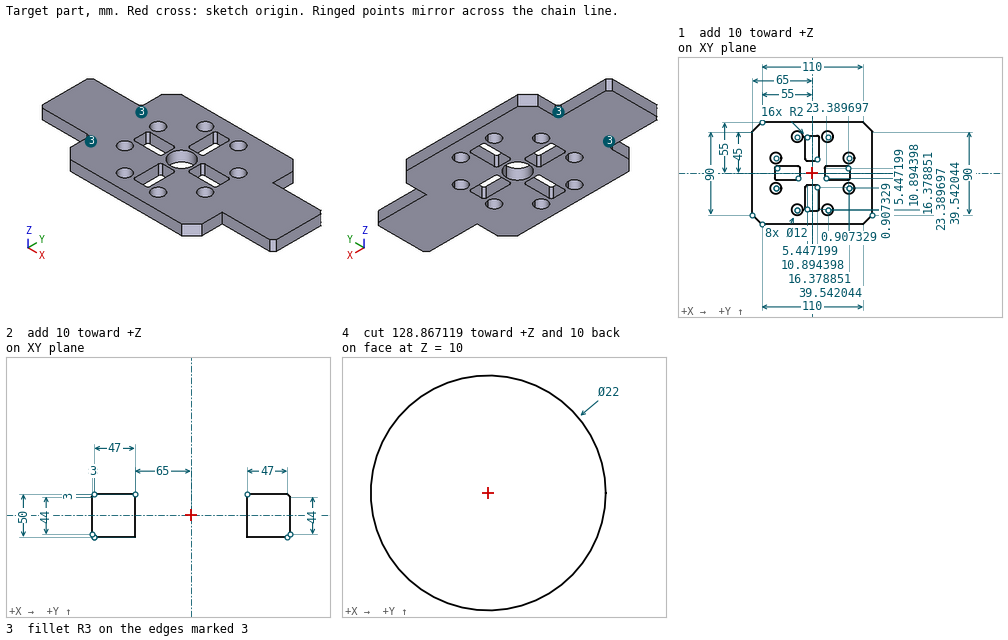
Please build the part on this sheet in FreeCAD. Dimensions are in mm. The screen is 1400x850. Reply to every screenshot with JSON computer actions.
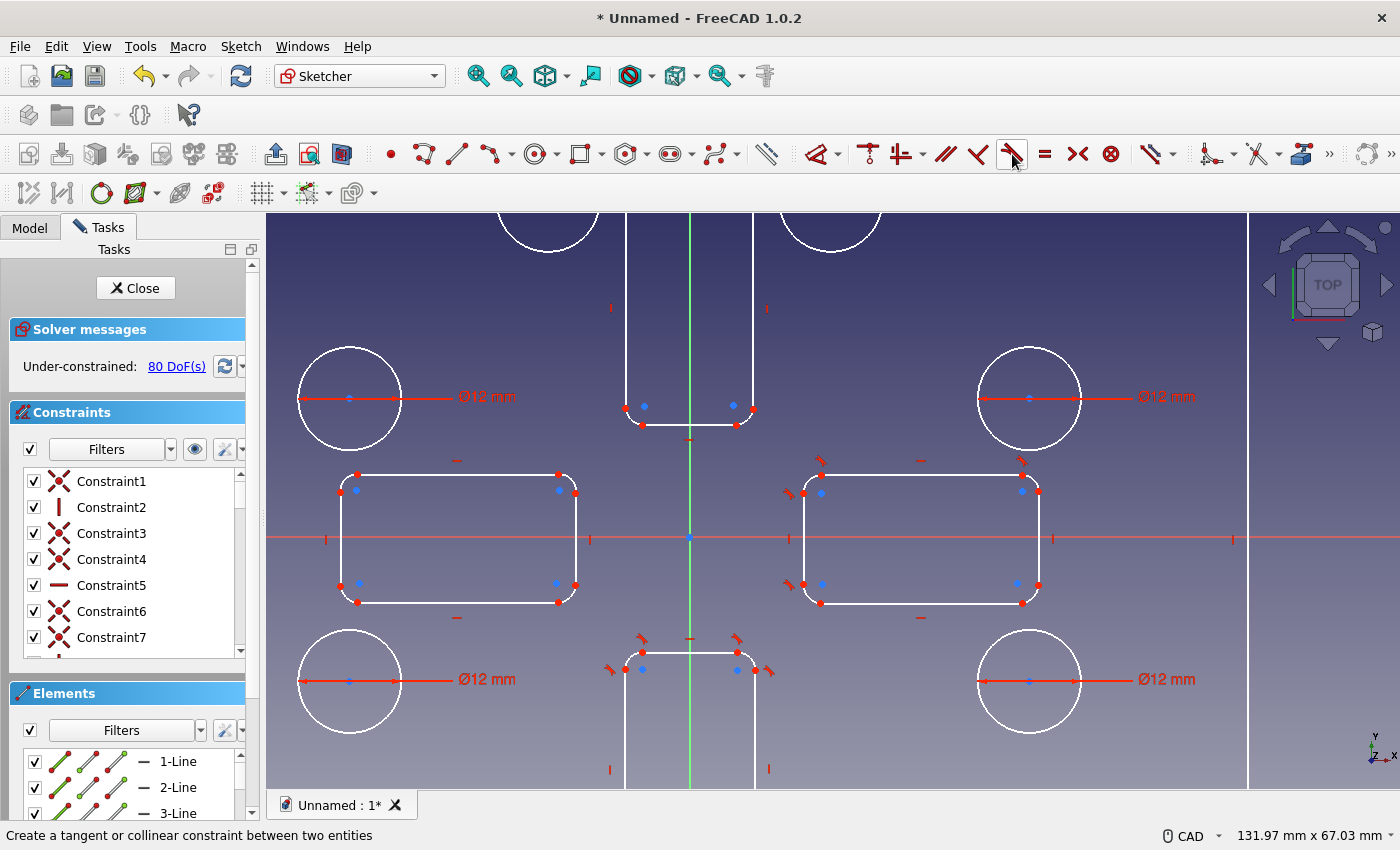
{"action": "left_click", "coordinate": [1039, 520]}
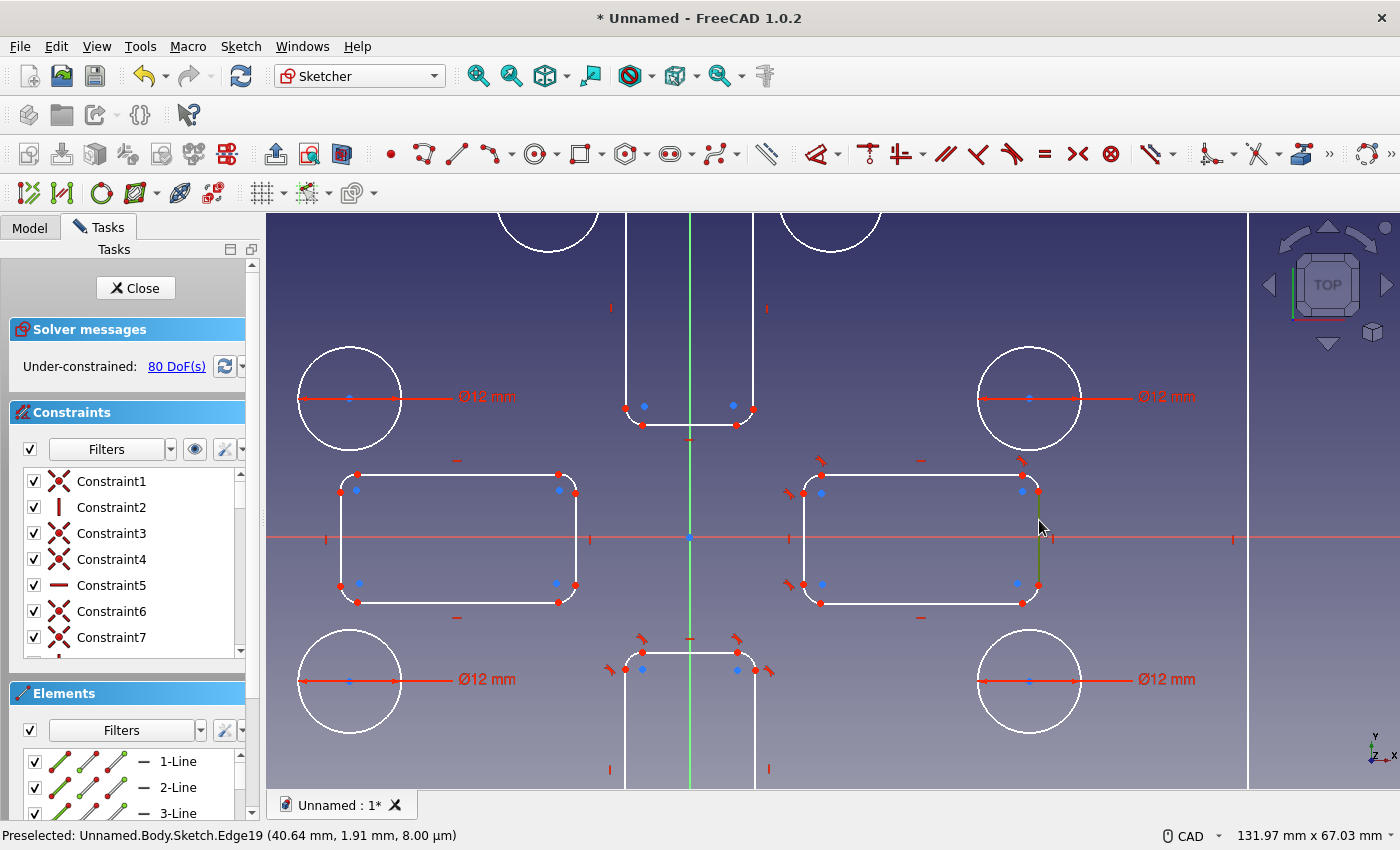
{"action": "left_click", "coordinate": [1034, 480]}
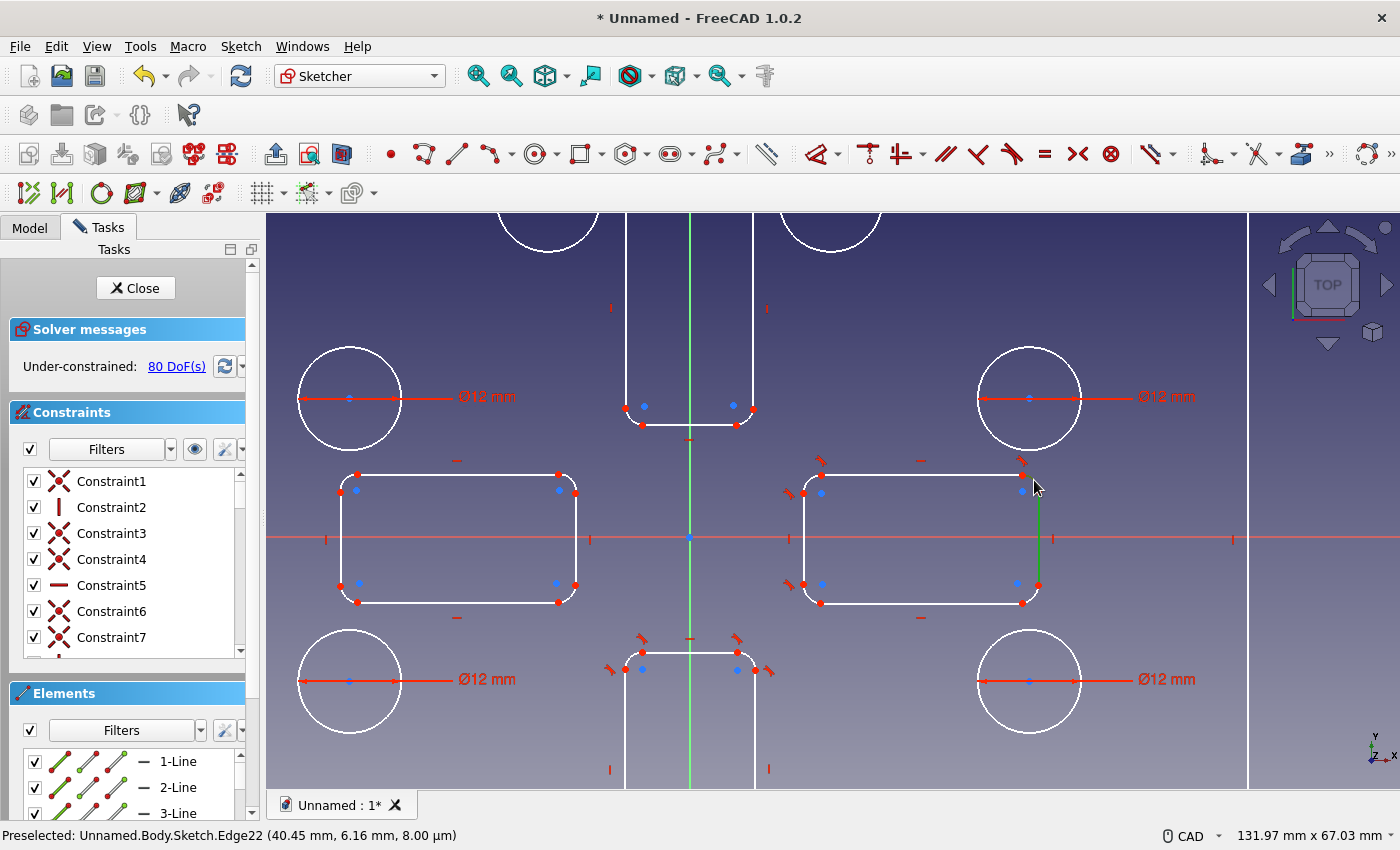
{"action": "left_click", "coordinate": [1012, 154]}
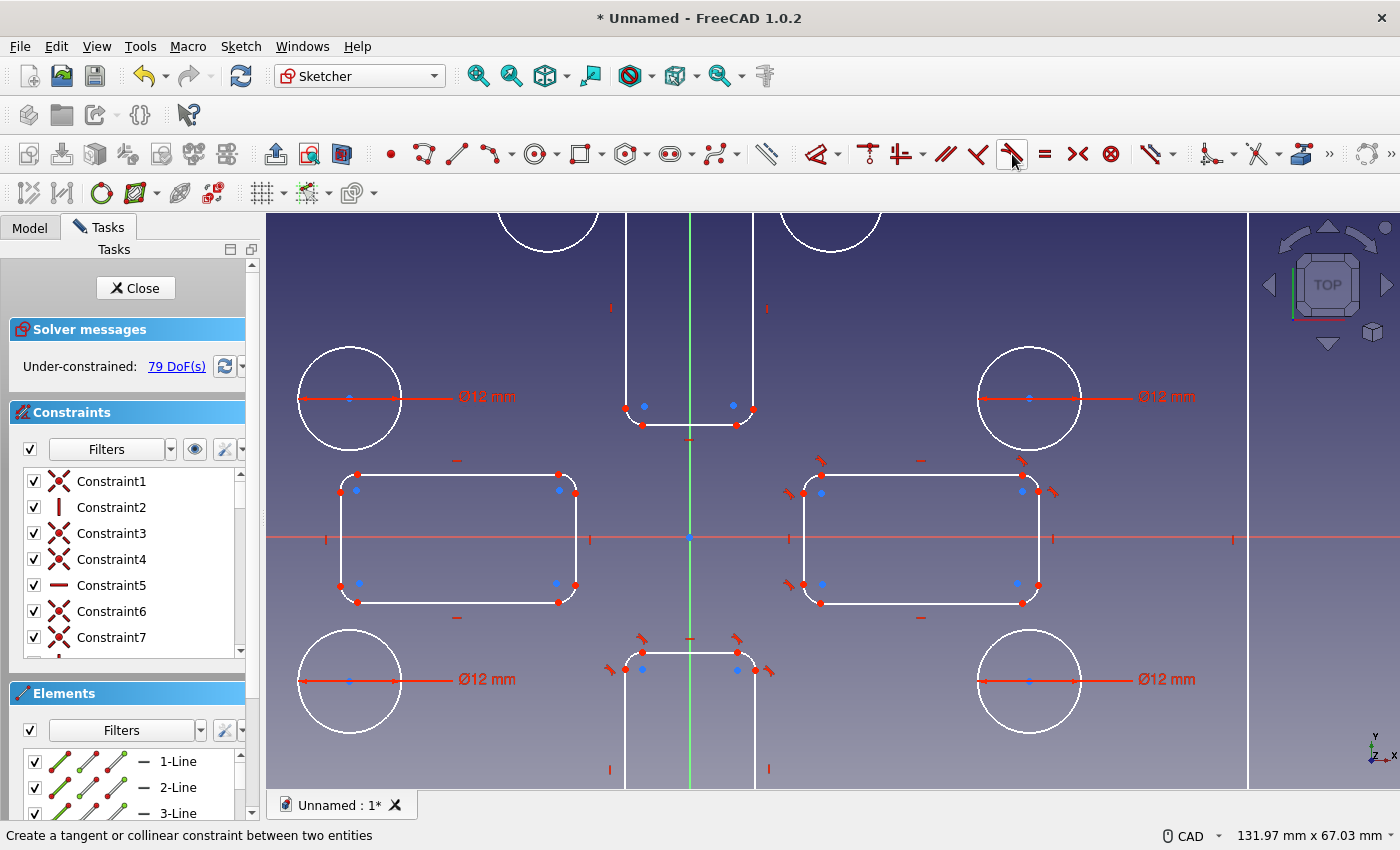
{"action": "left_click", "coordinate": [1039, 520]}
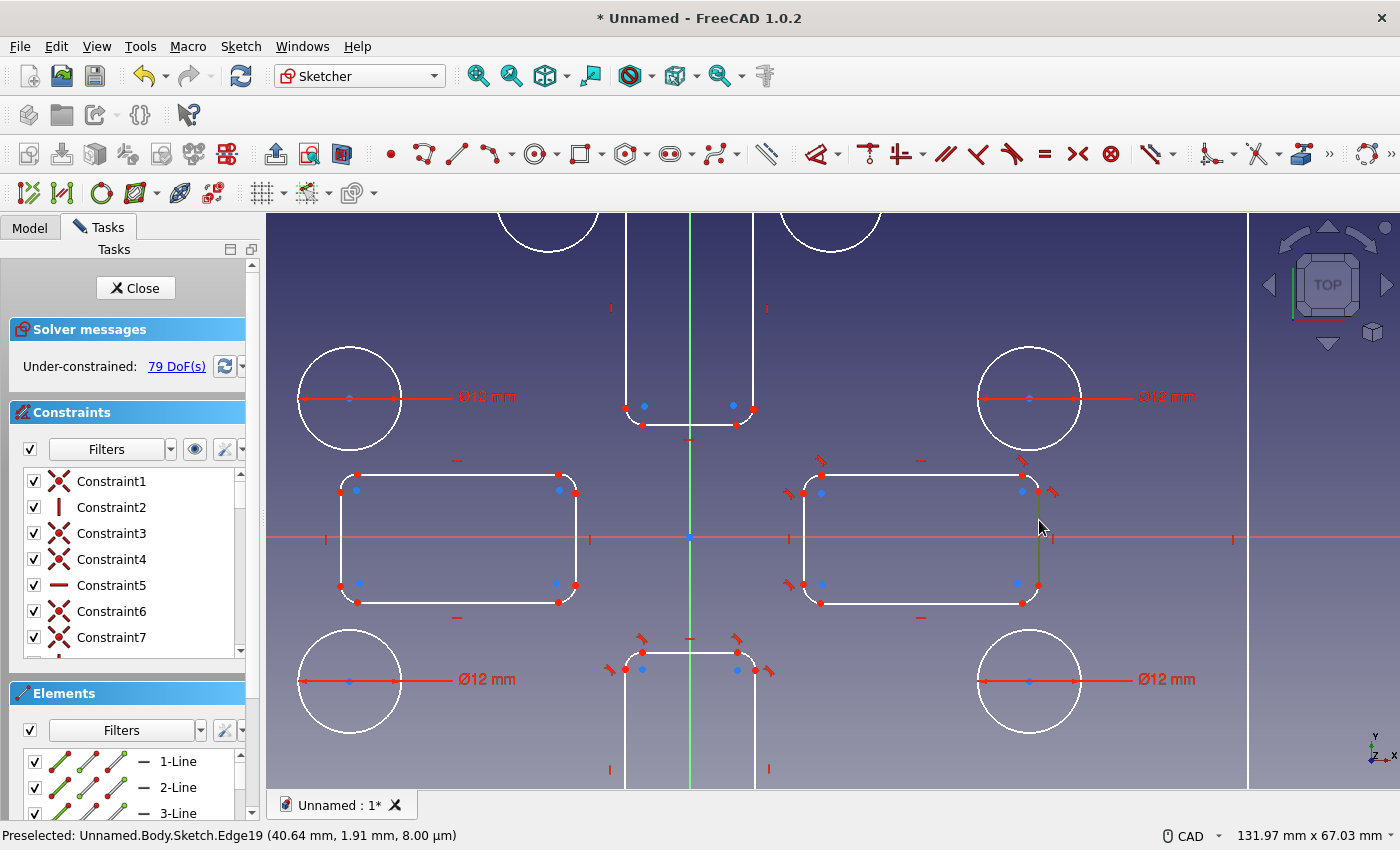
{"action": "left_click", "coordinate": [1033, 597]}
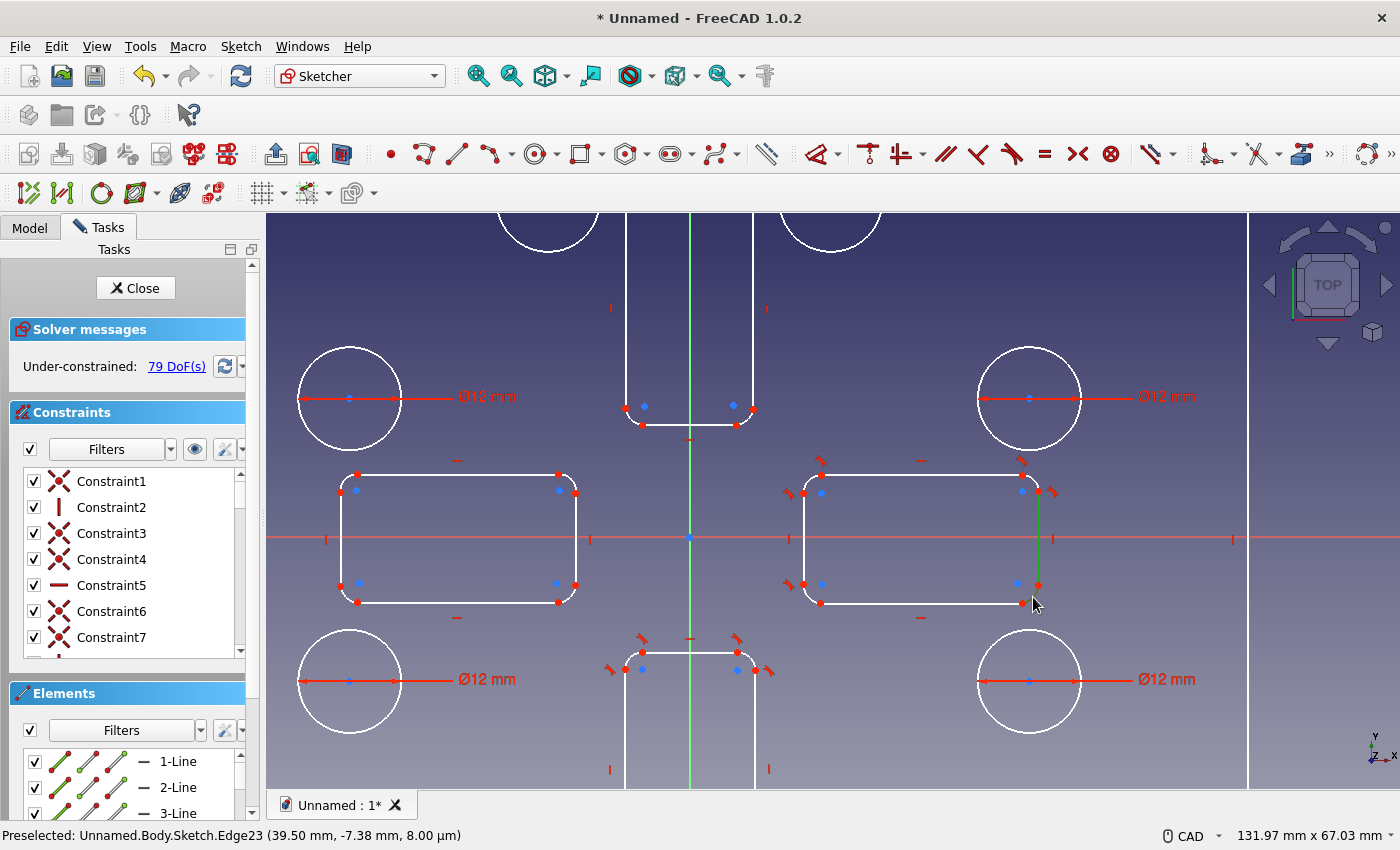
{"action": "left_click", "coordinate": [1012, 154]}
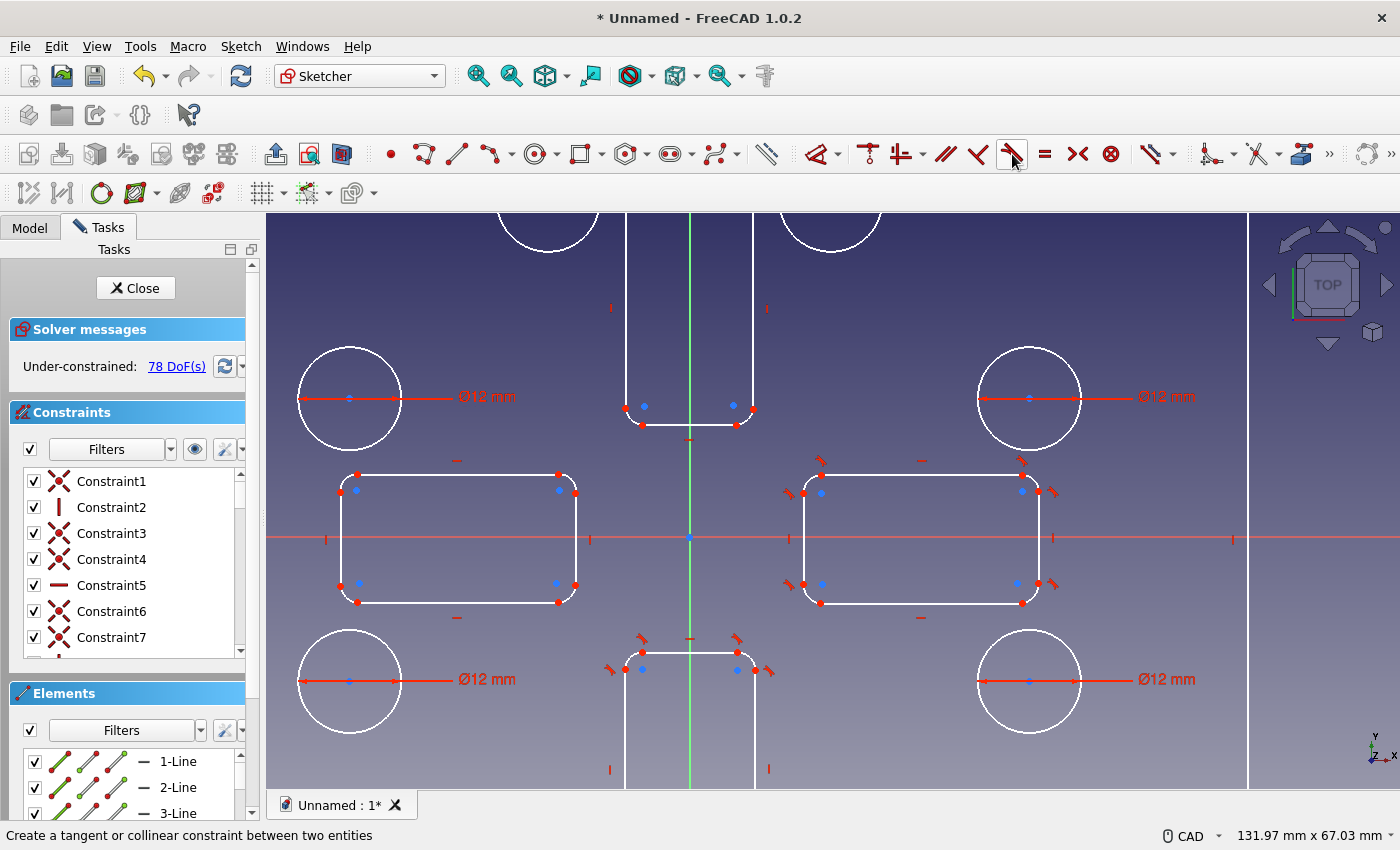
{"action": "left_click", "coordinate": [962, 604]}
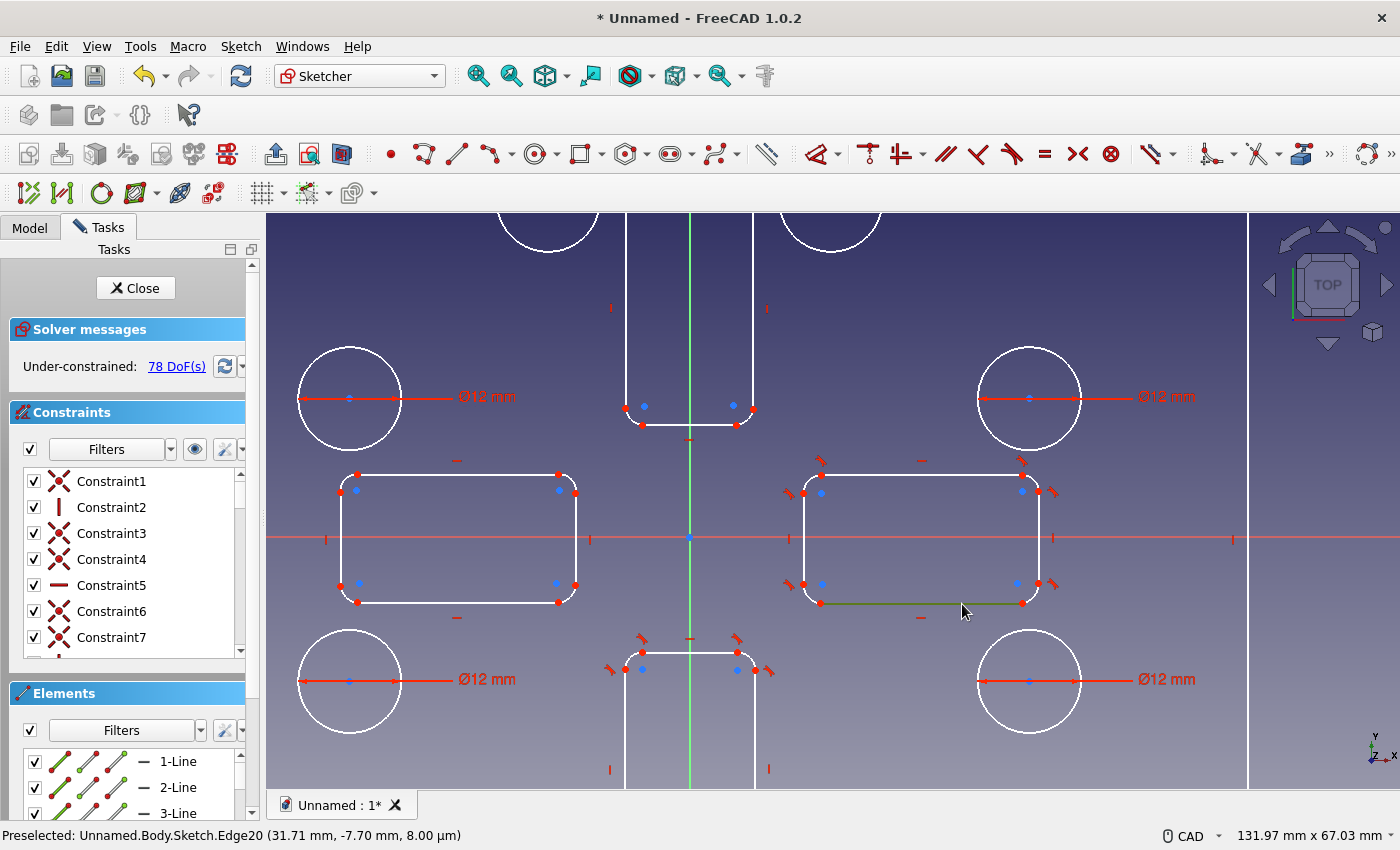
{"action": "left_click", "coordinate": [1034, 596]}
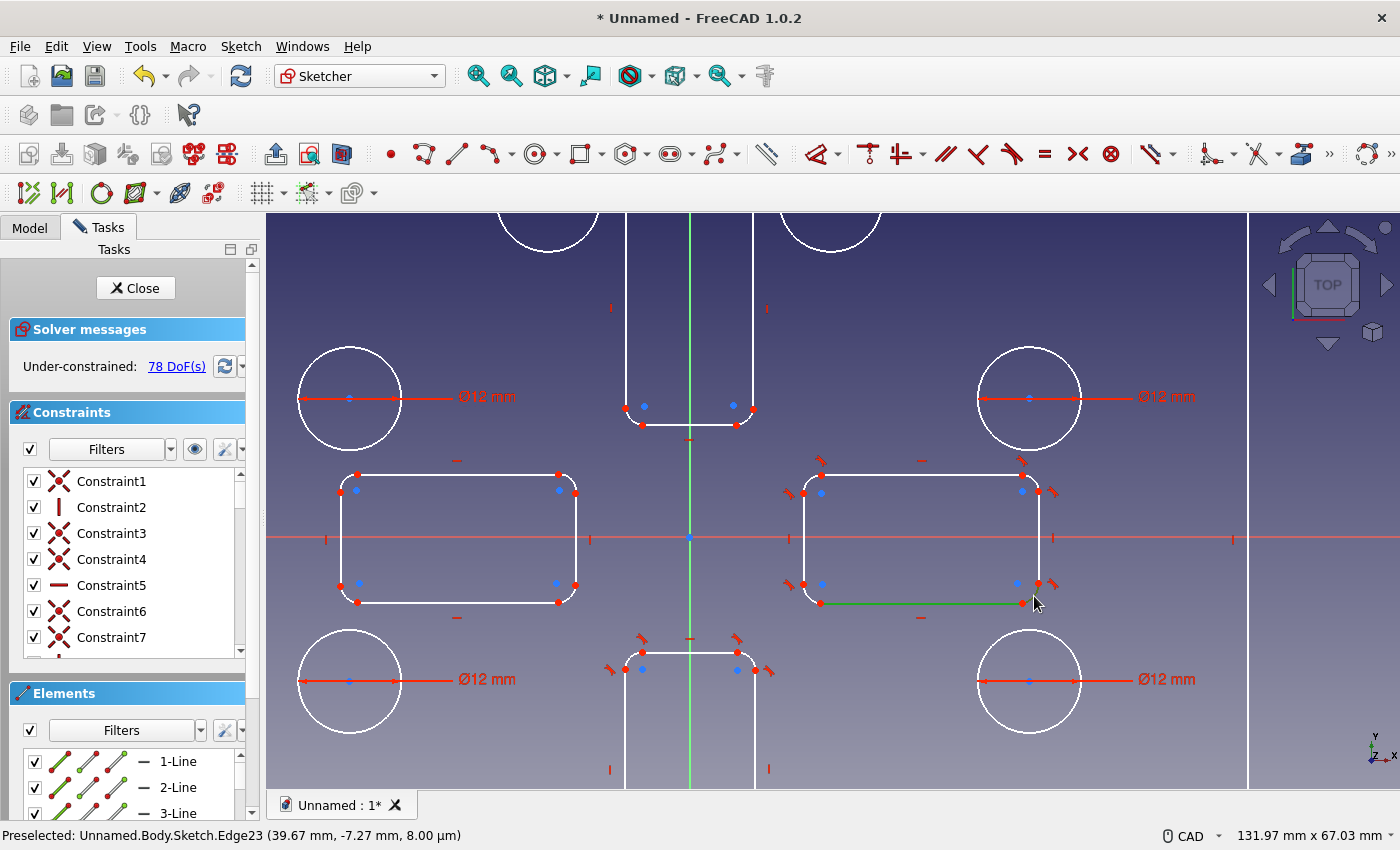
{"action": "left_click", "coordinate": [1012, 154]}